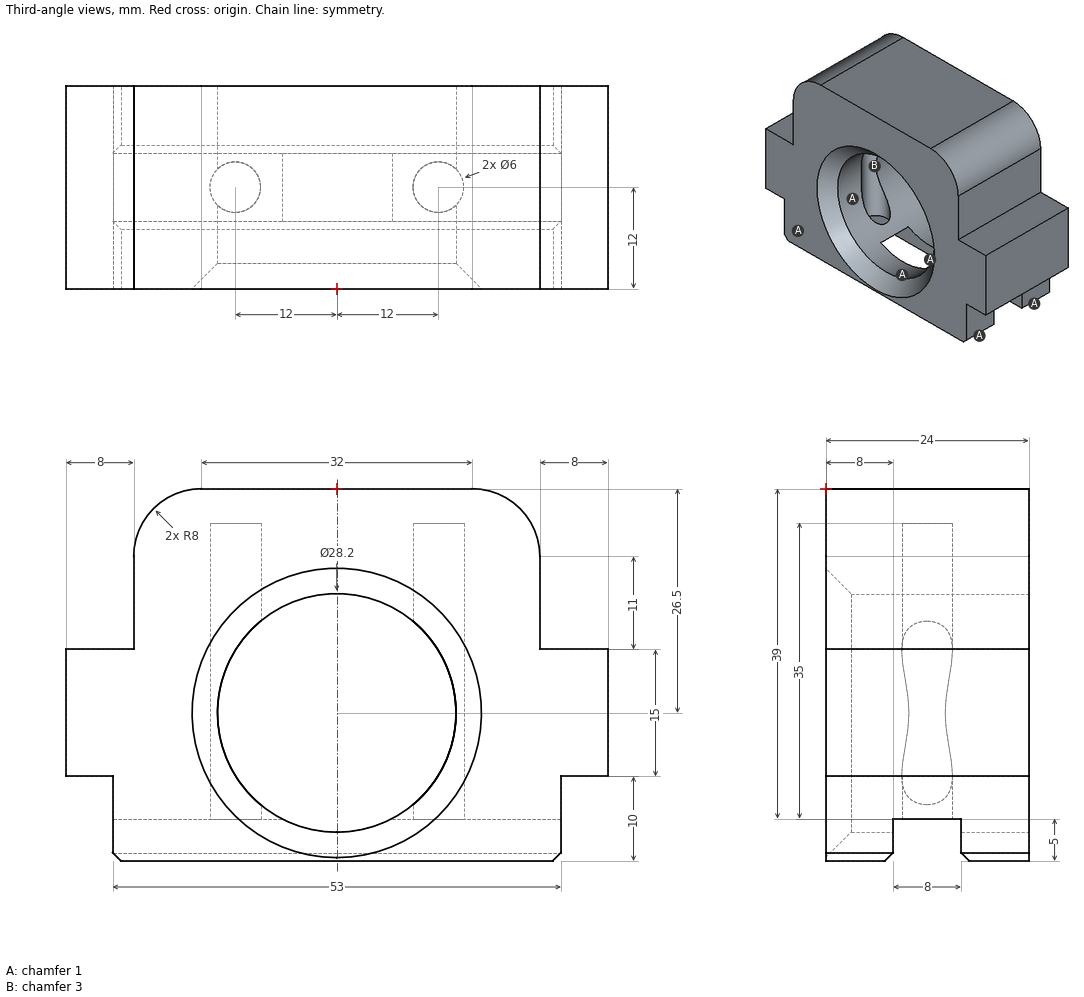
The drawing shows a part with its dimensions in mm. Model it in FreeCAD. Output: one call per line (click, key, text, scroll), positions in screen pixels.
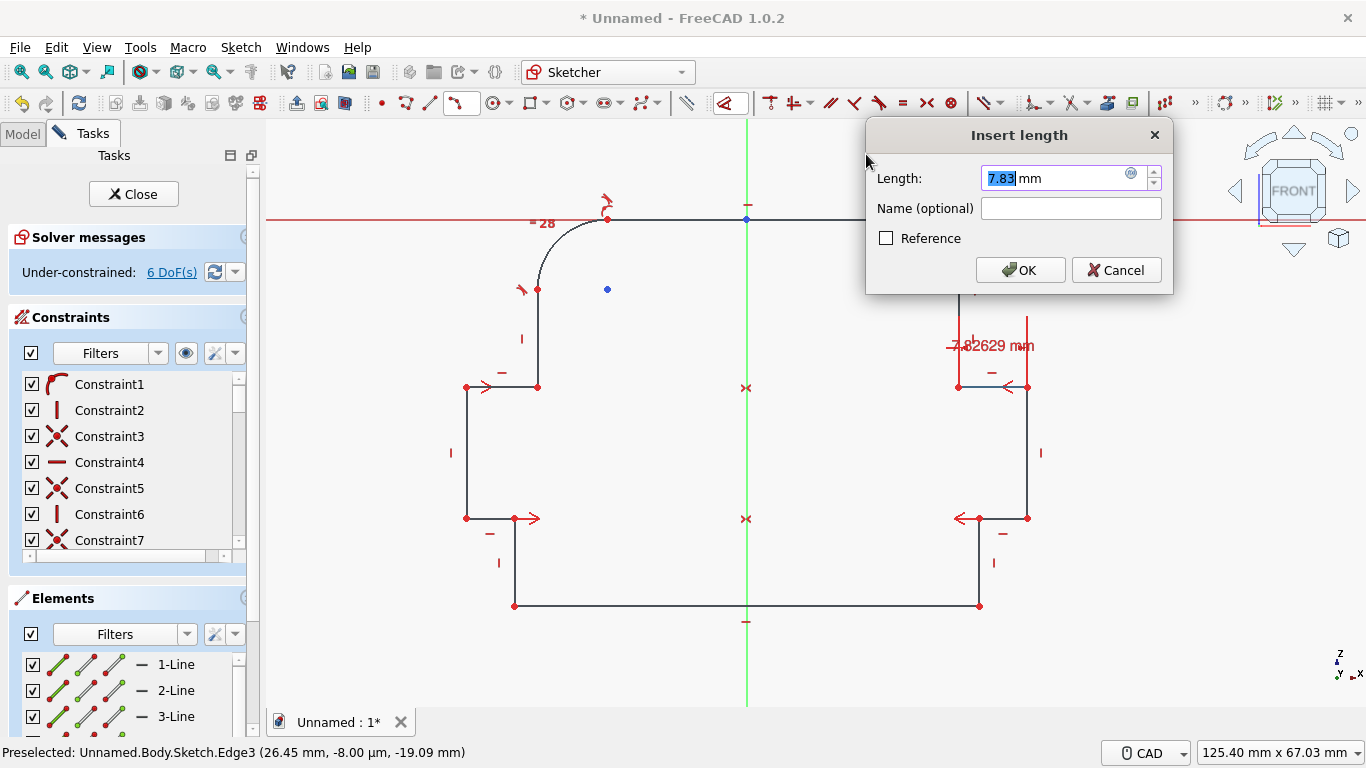
text(8)
key(Return)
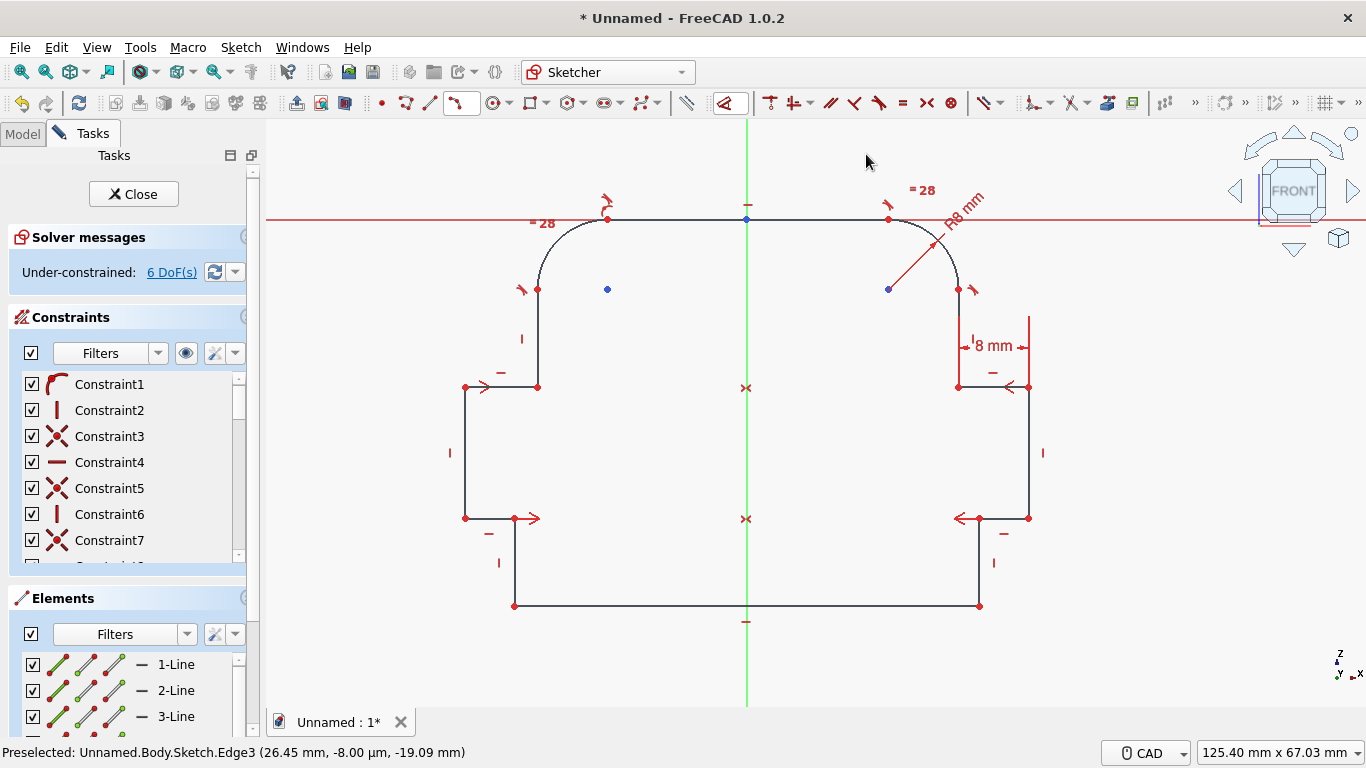
click(516, 387)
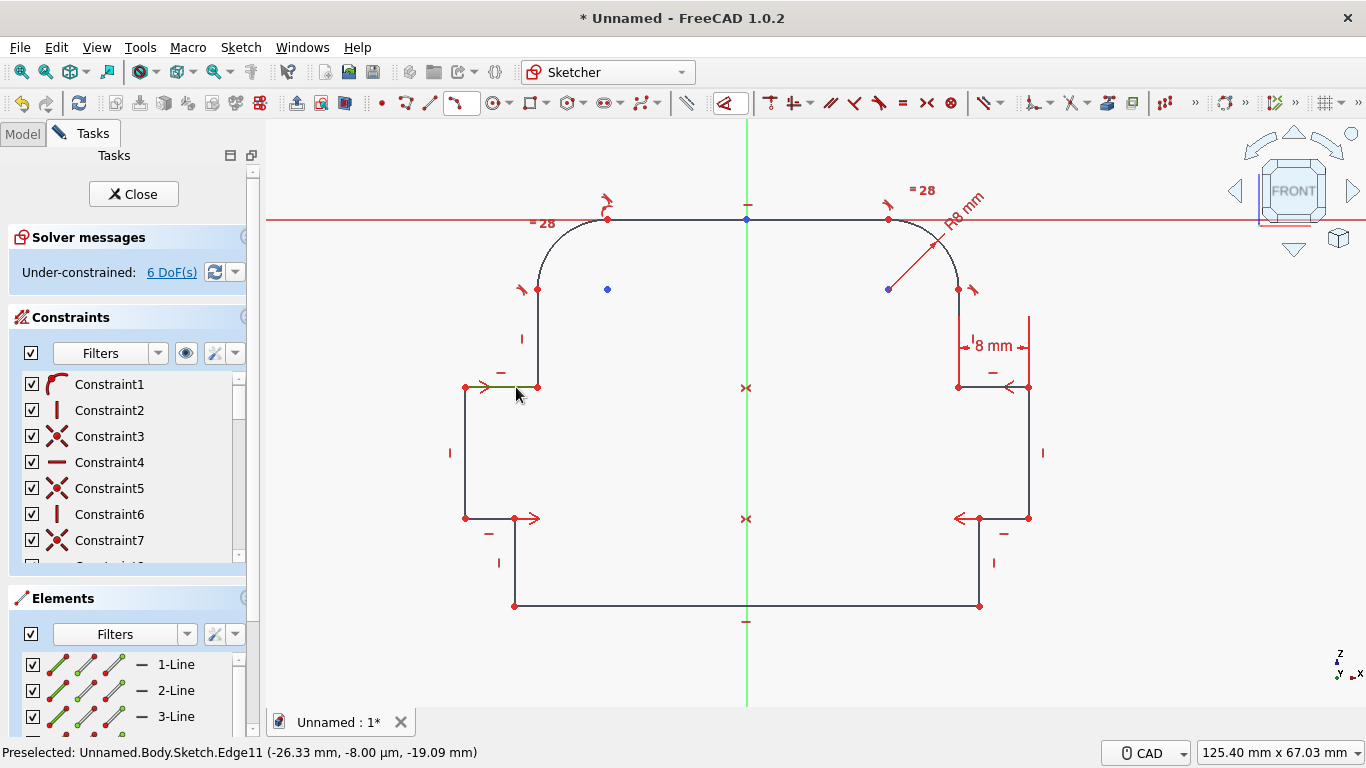
key(l)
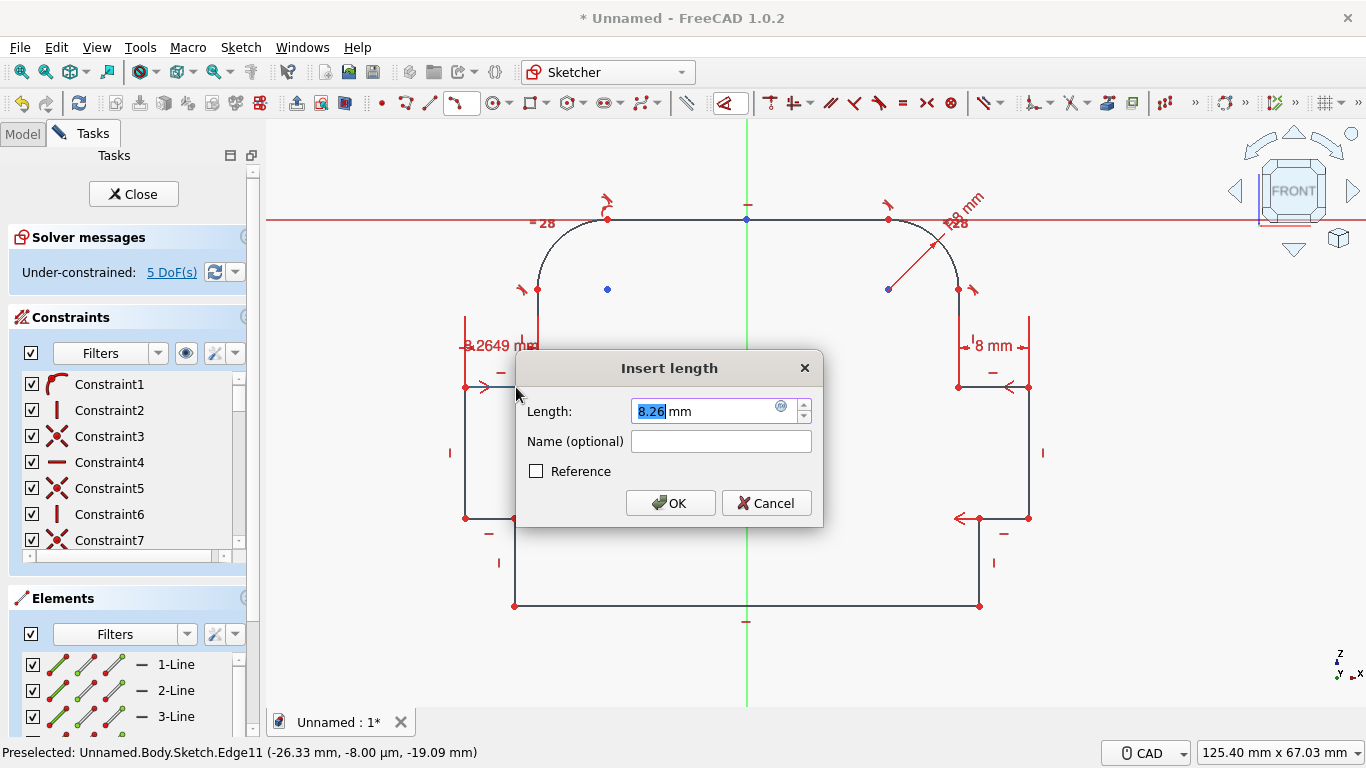
text(8)
key(Return)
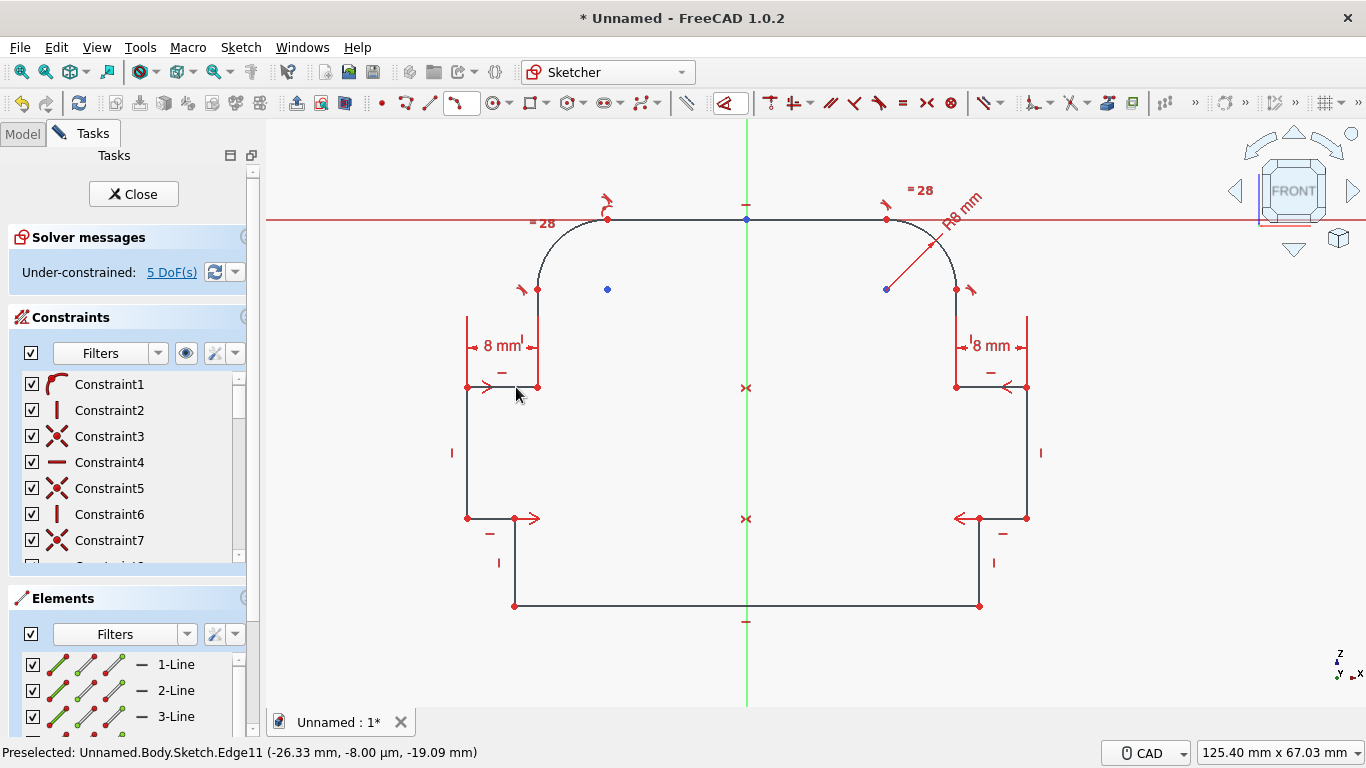
click(691, 220)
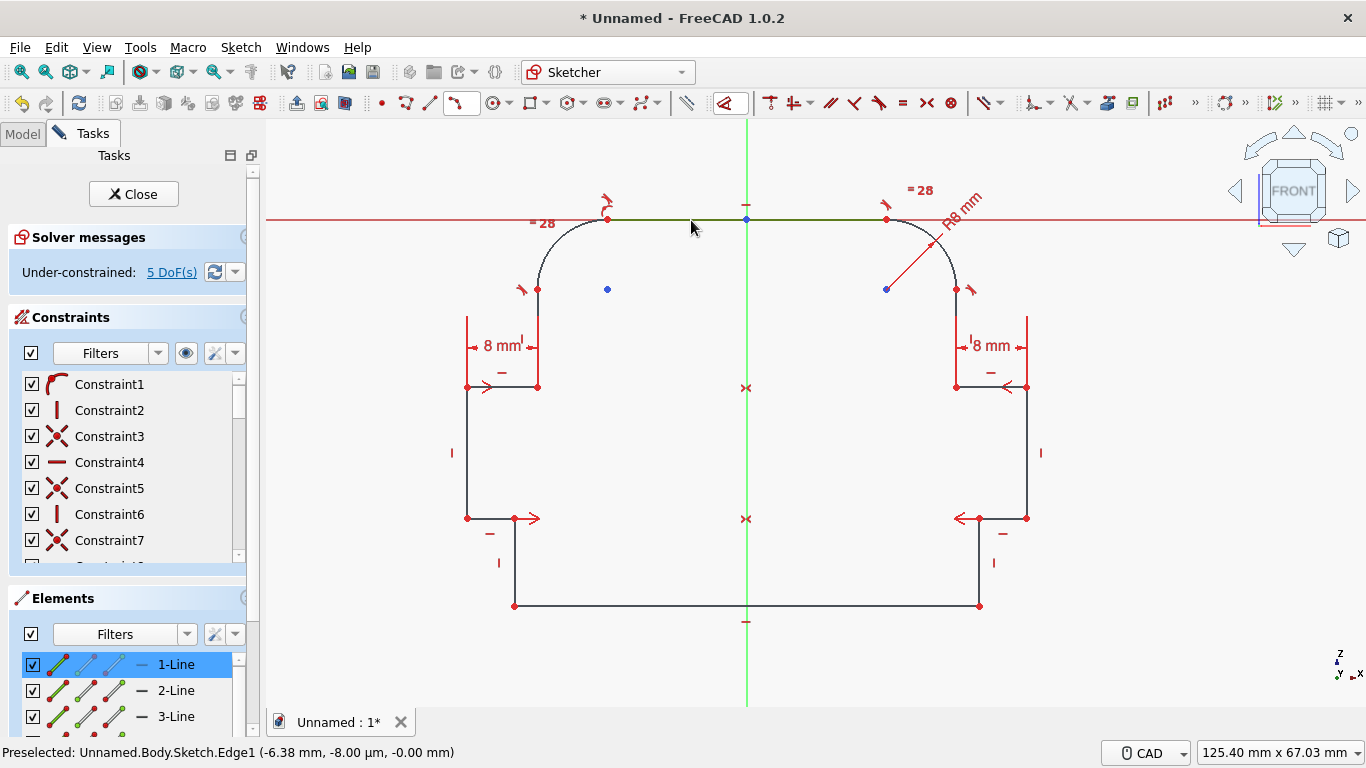
key(l)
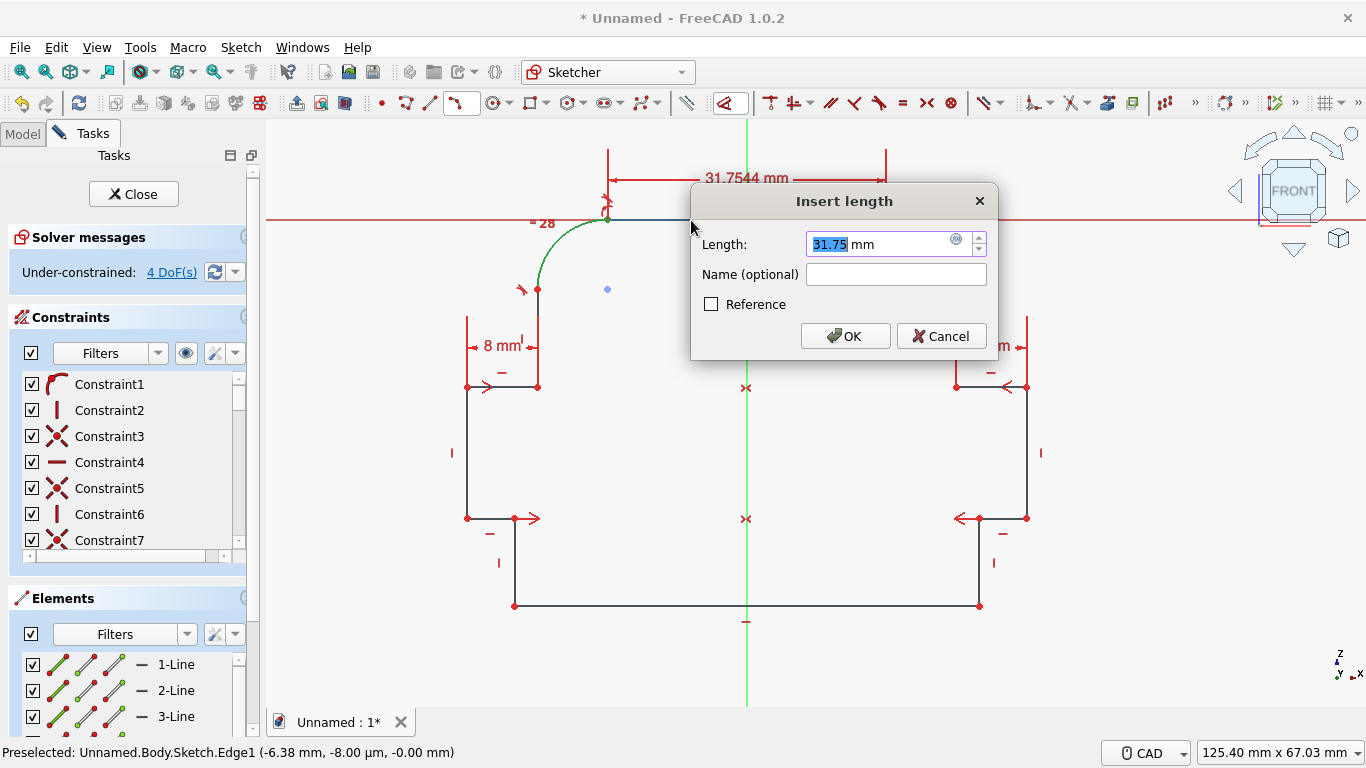
text(32)
key(Return)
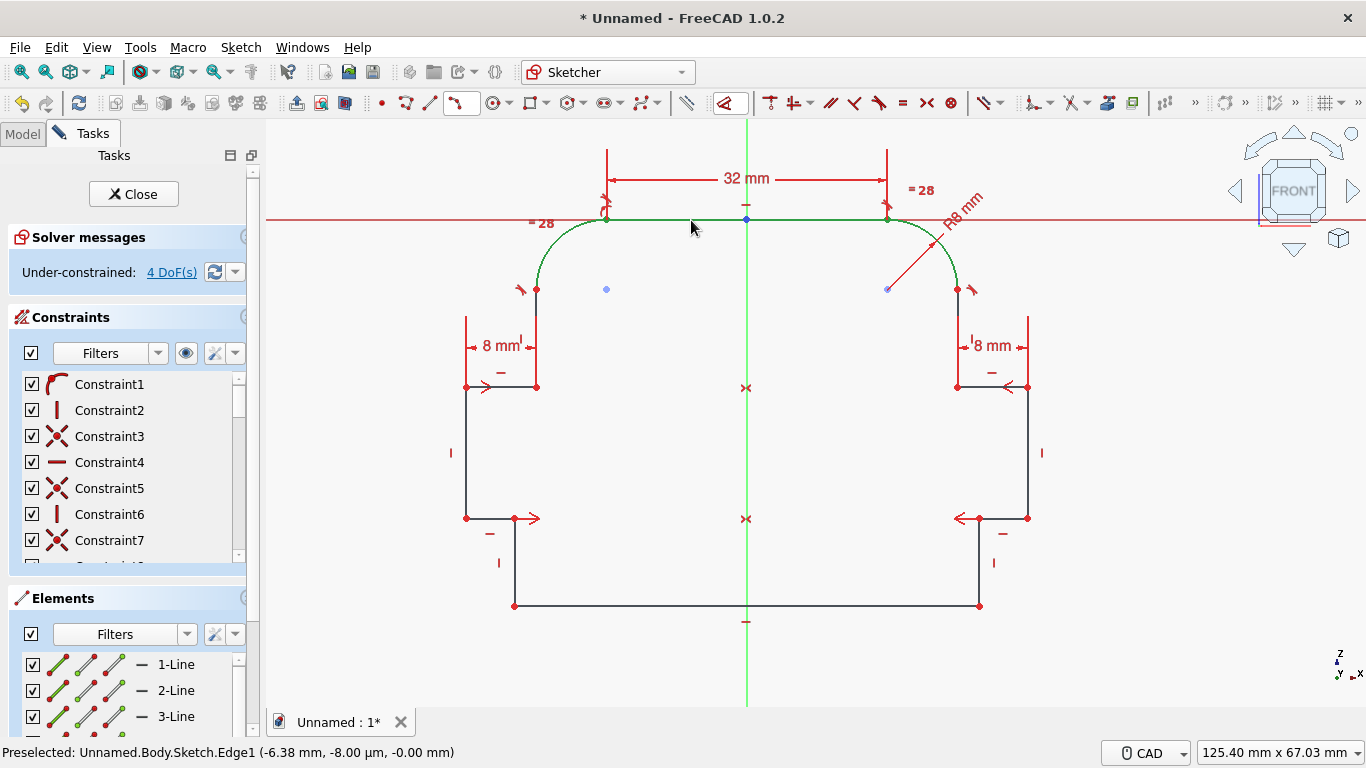
click(958, 319)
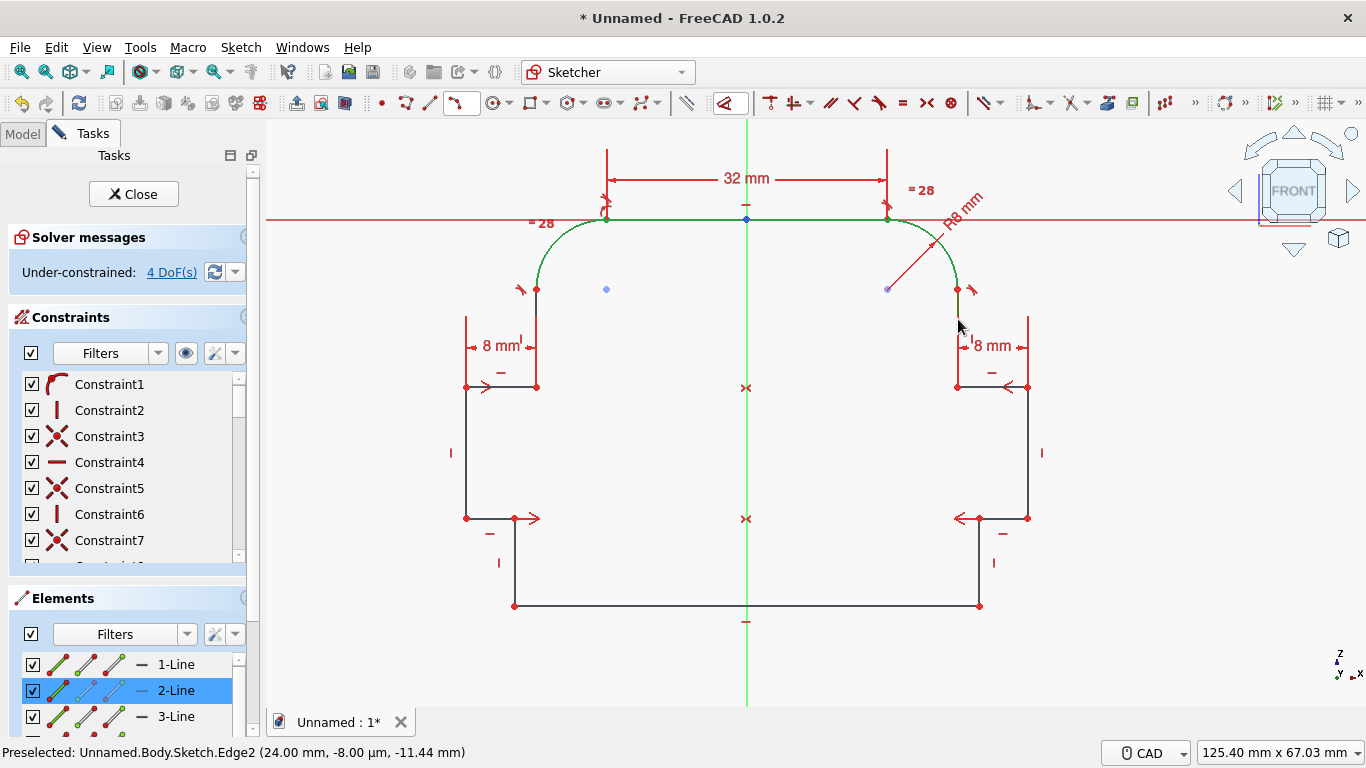
key(i)